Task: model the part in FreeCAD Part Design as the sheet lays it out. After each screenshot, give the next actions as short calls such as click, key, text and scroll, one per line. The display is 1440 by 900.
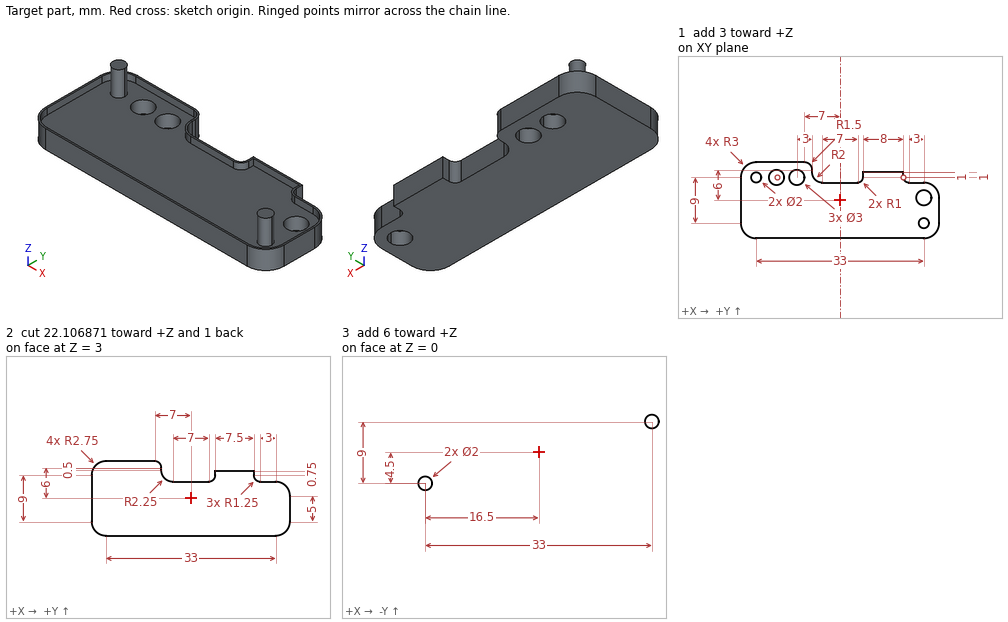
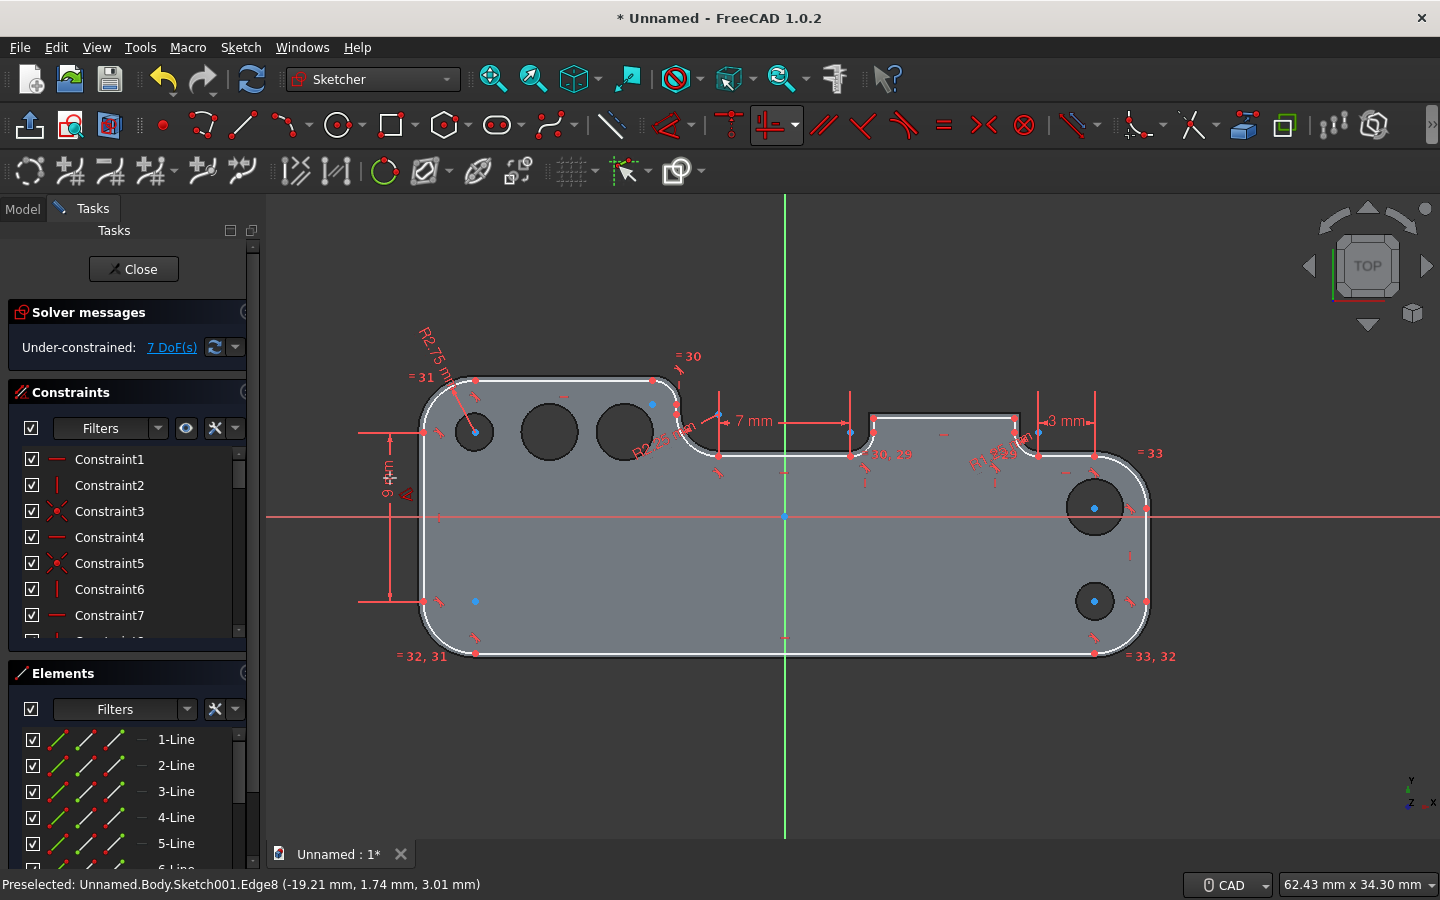
click(1147, 574)
click(1181, 555)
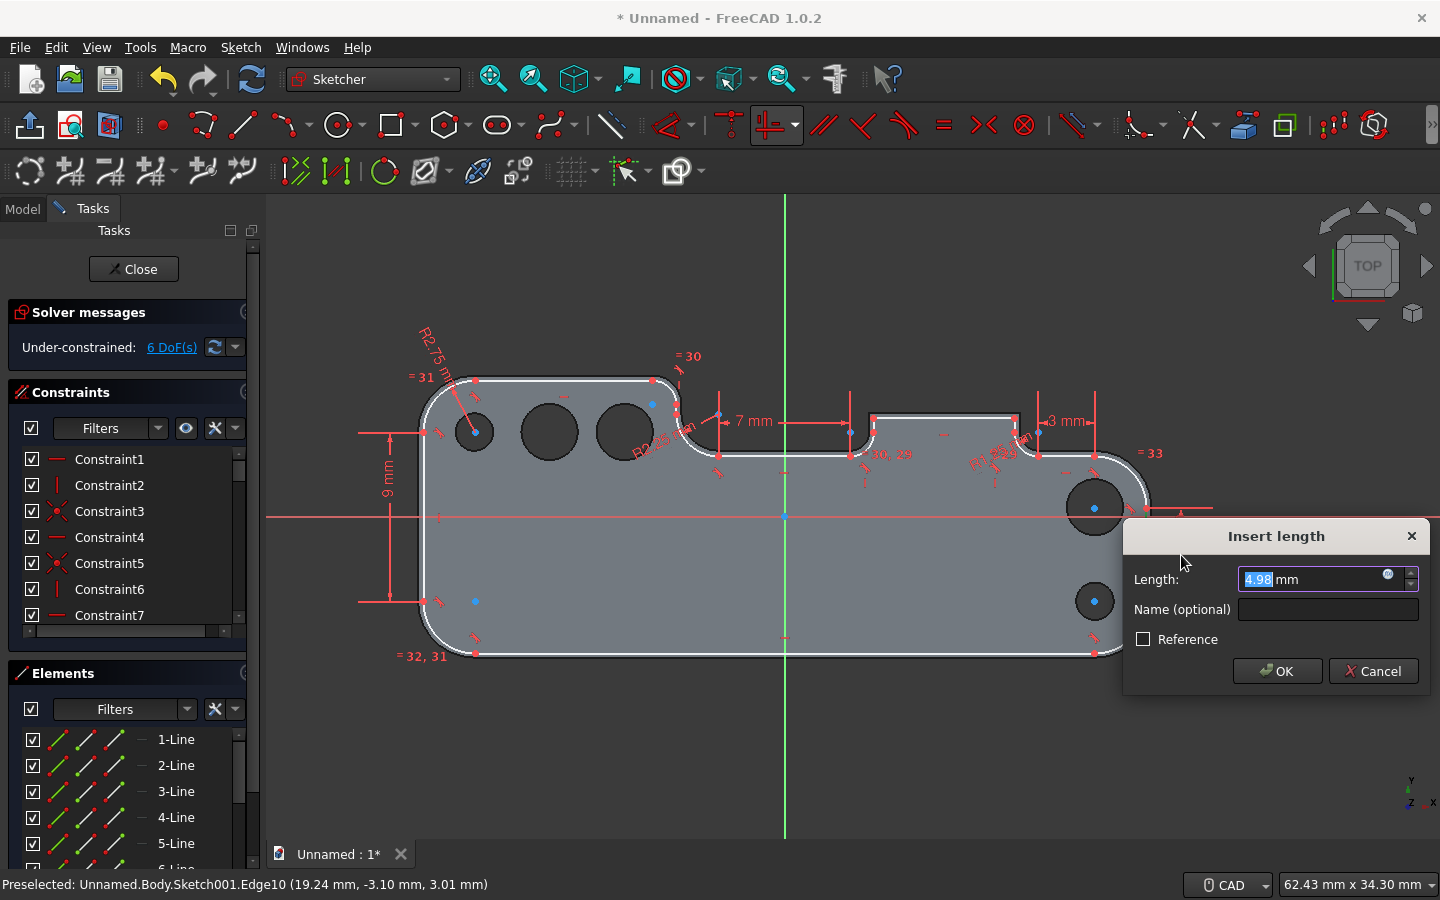
text(5)
key(Return)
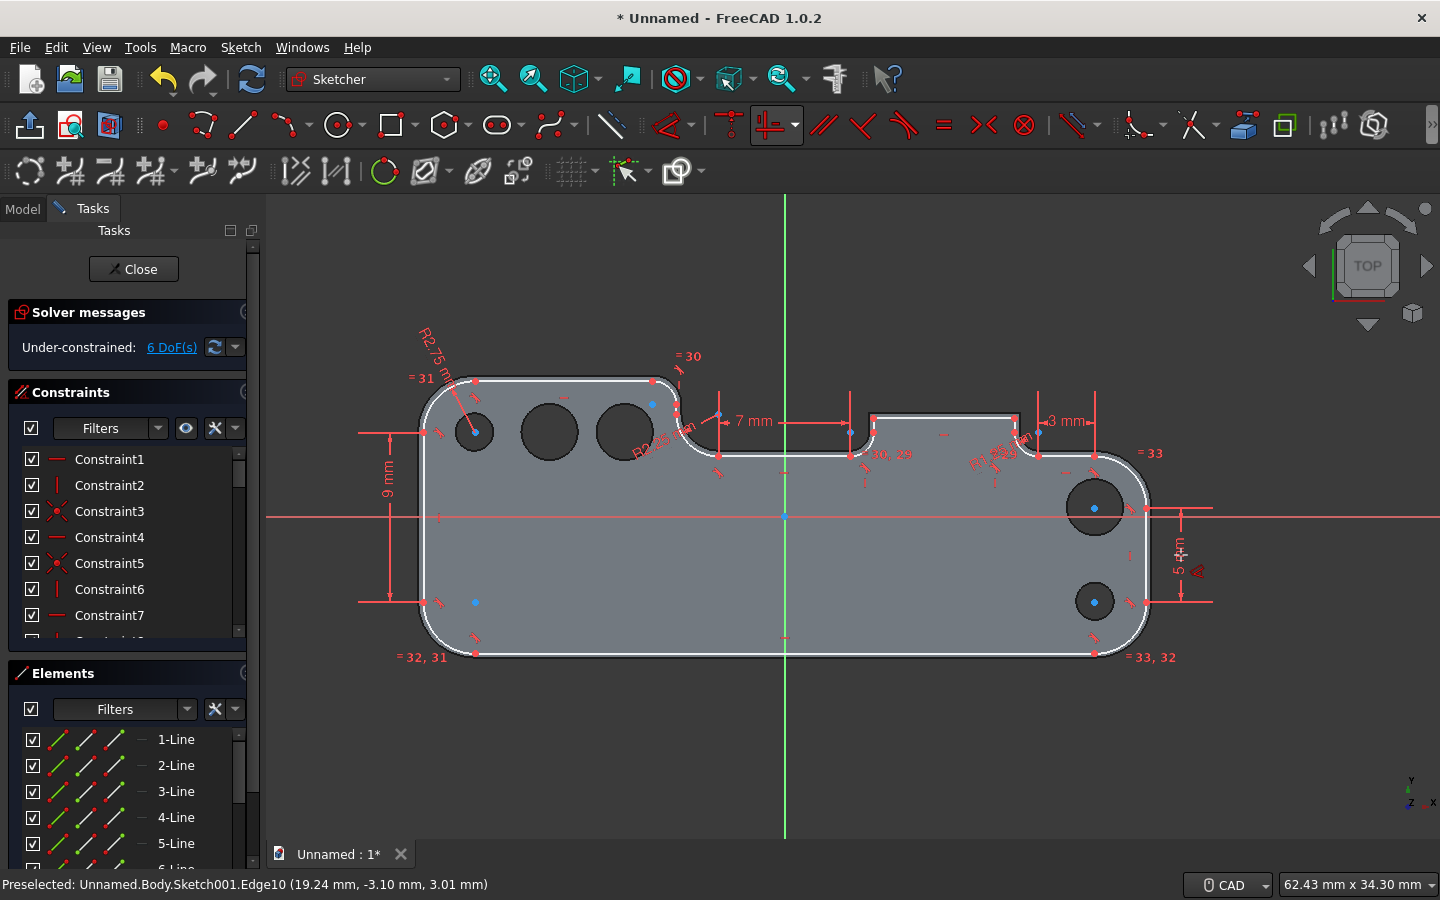
click(661, 654)
click(643, 688)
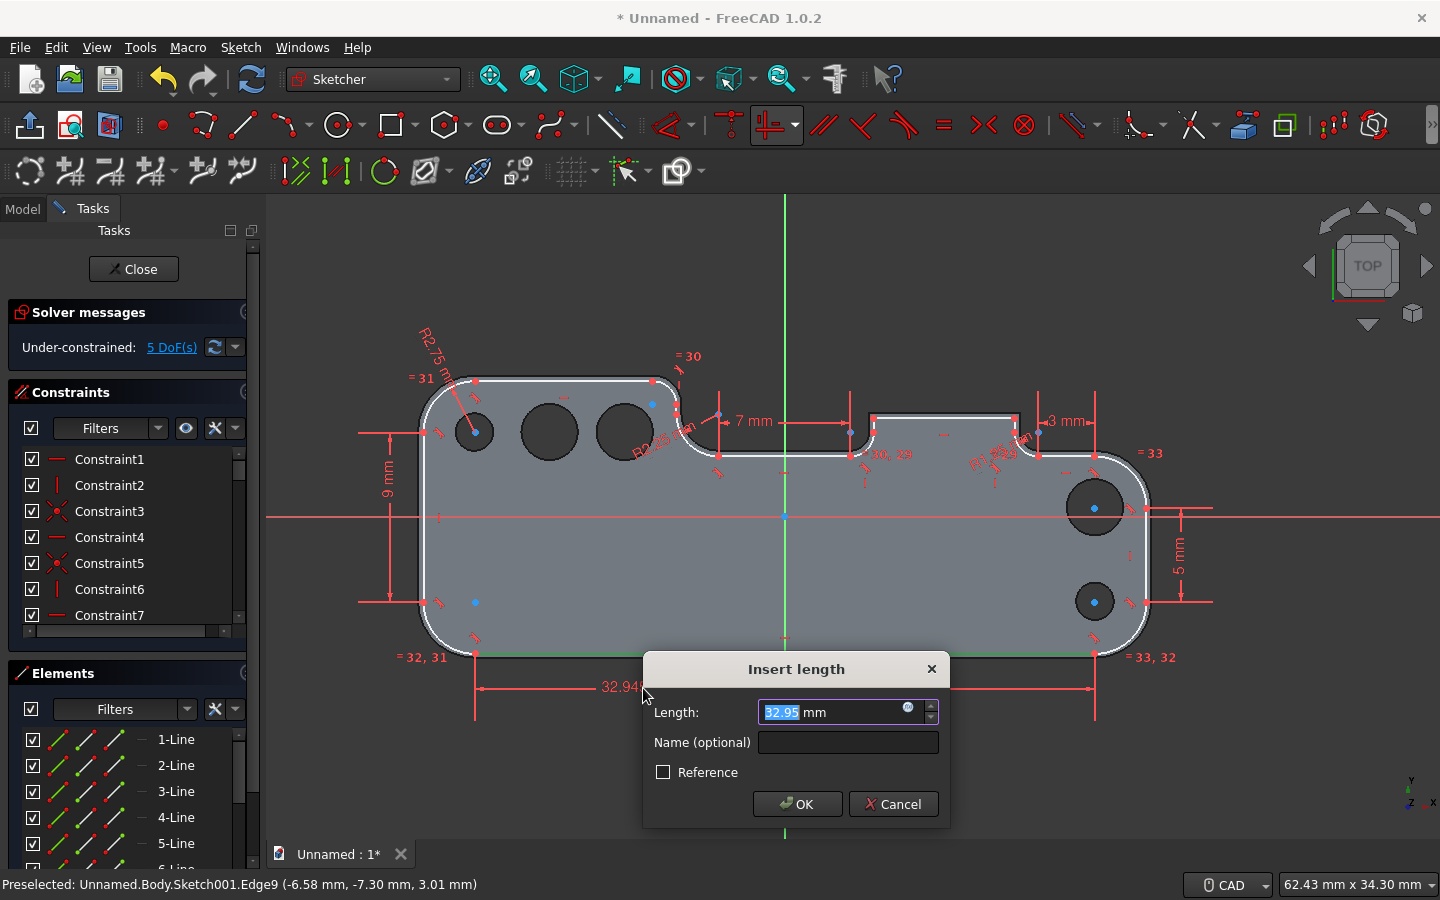
text(33)
key(Return)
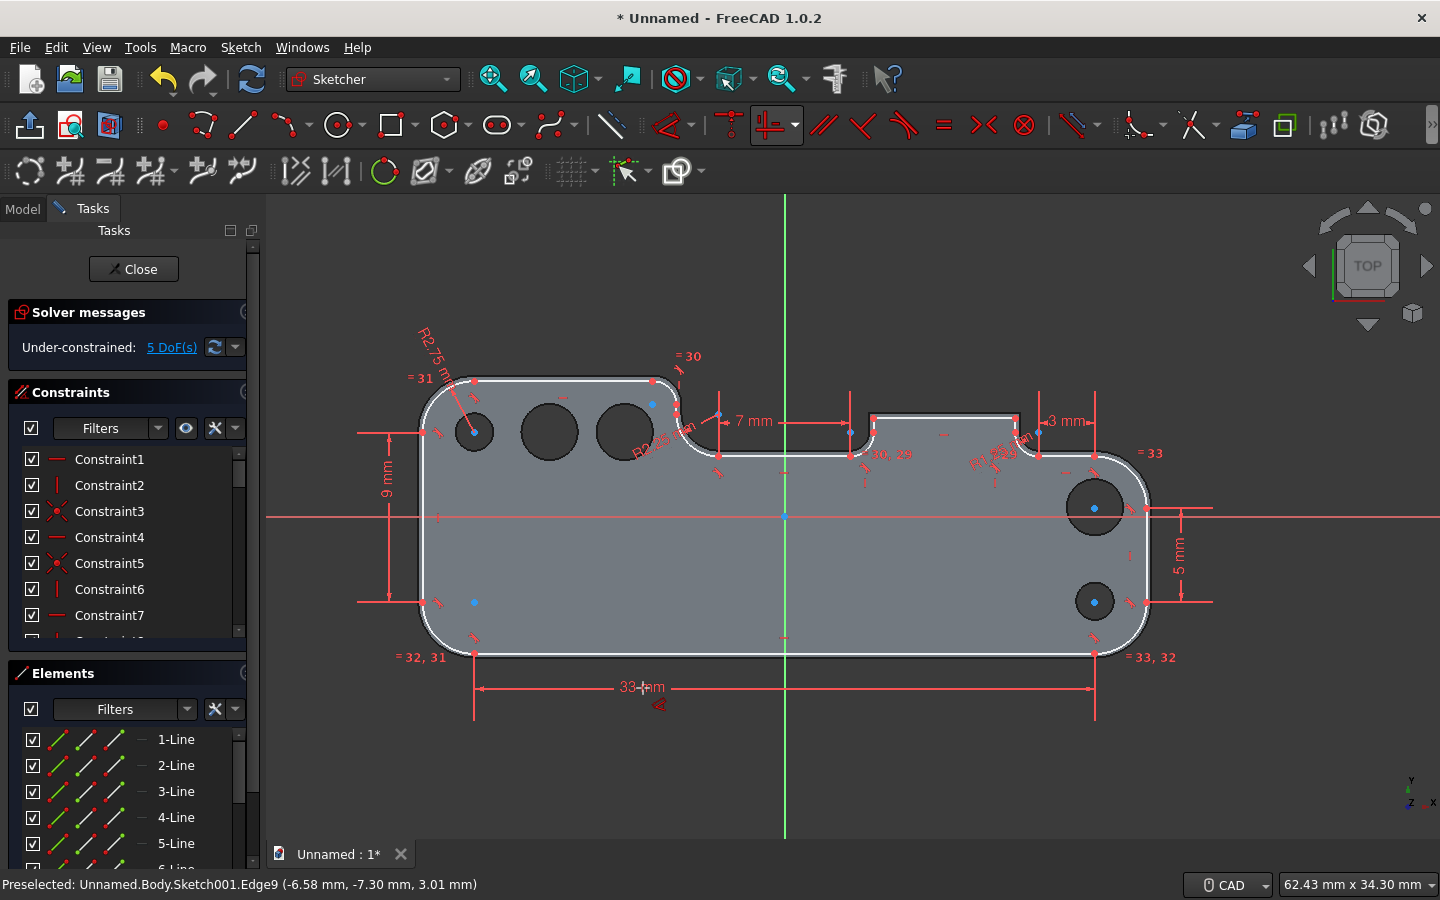
scroll(676, 405, up, 2)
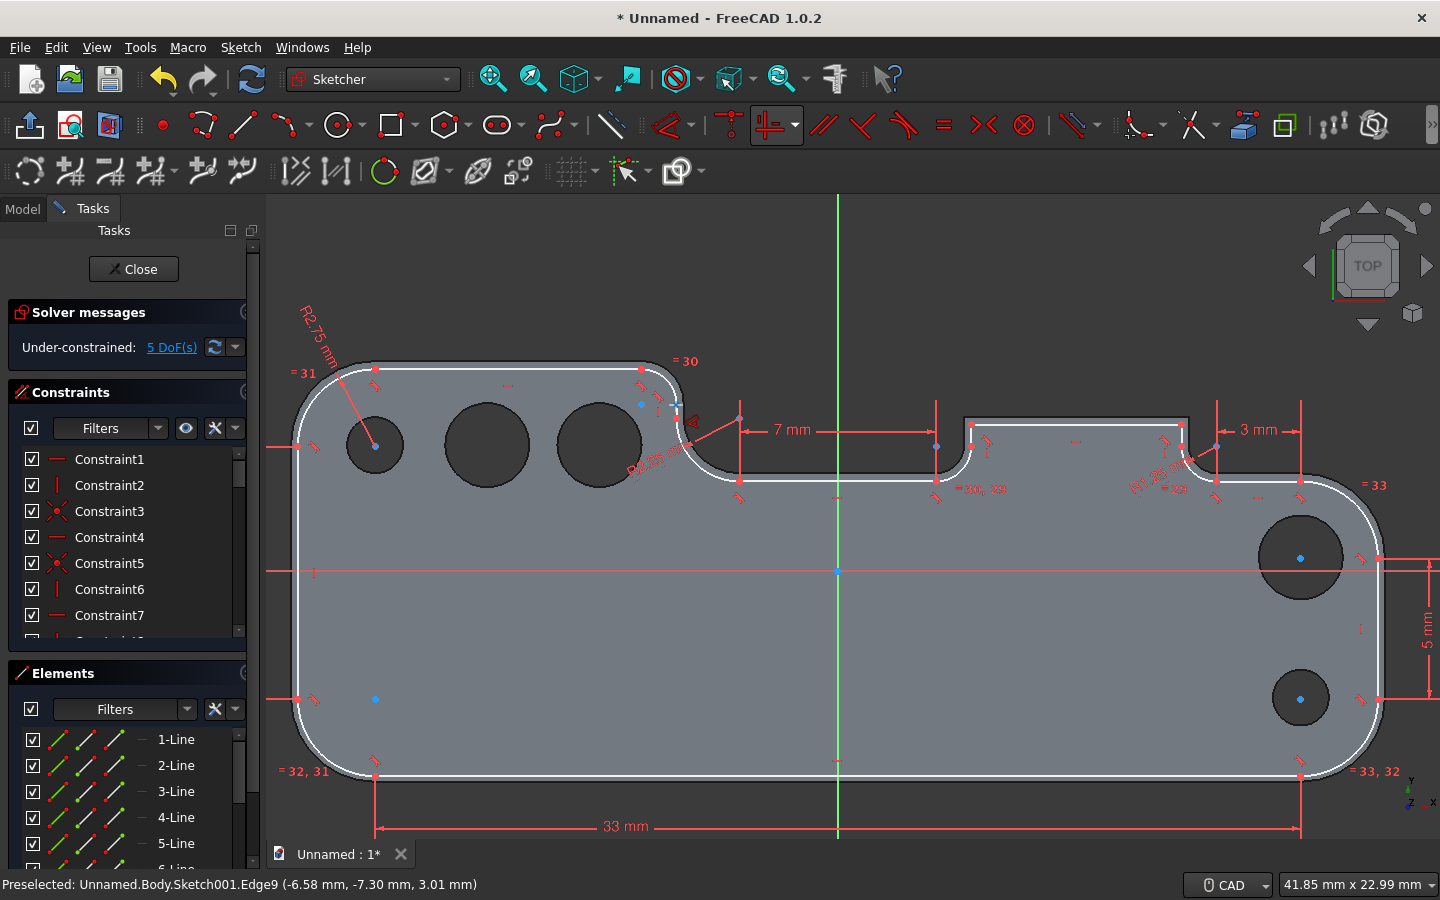
click(677, 404)
click(643, 488)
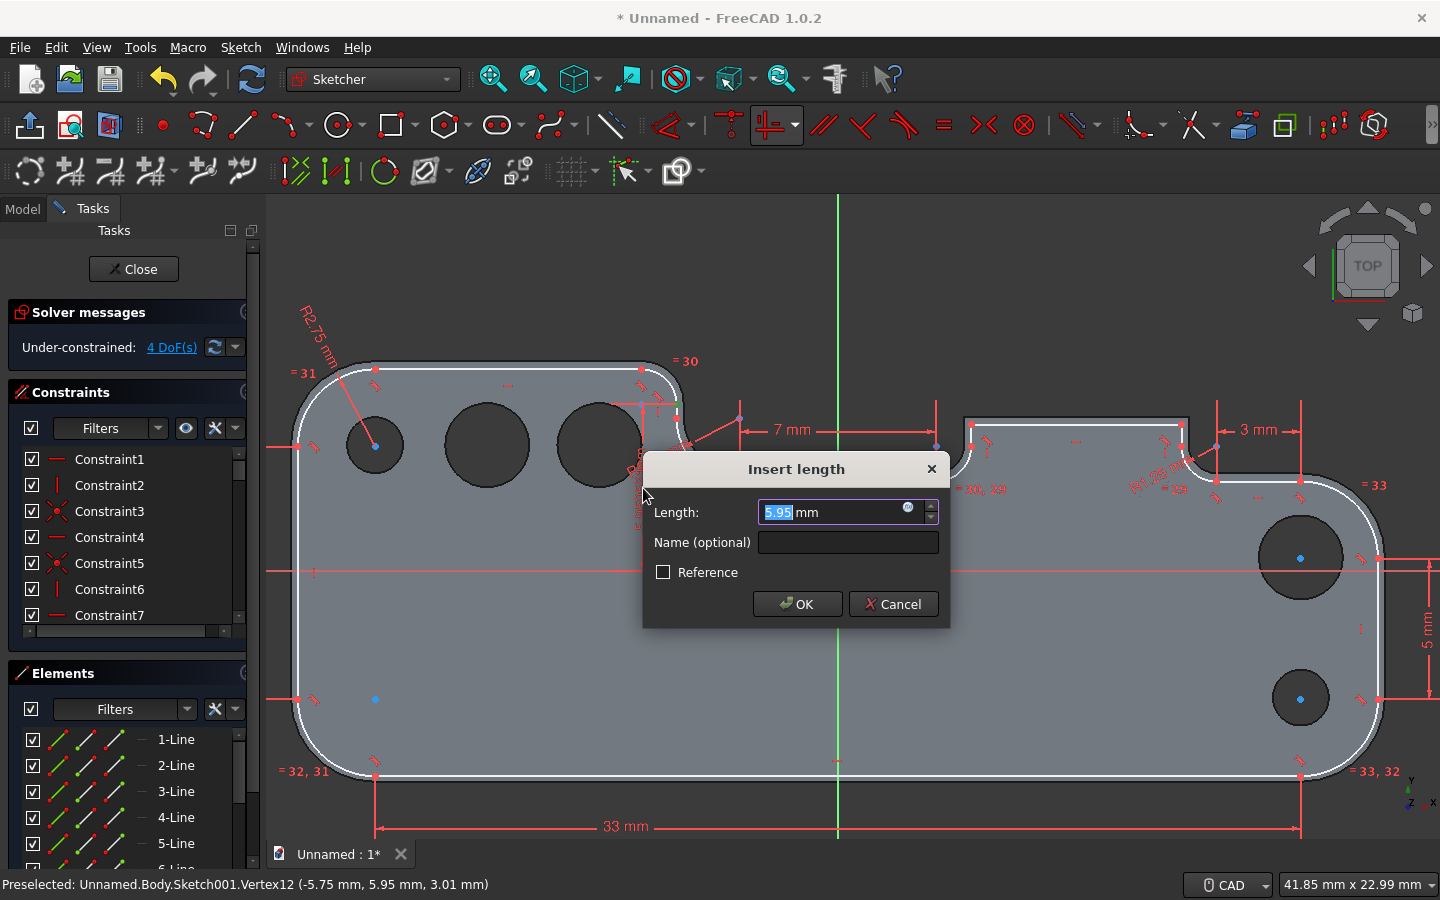
text(6)
key(Return)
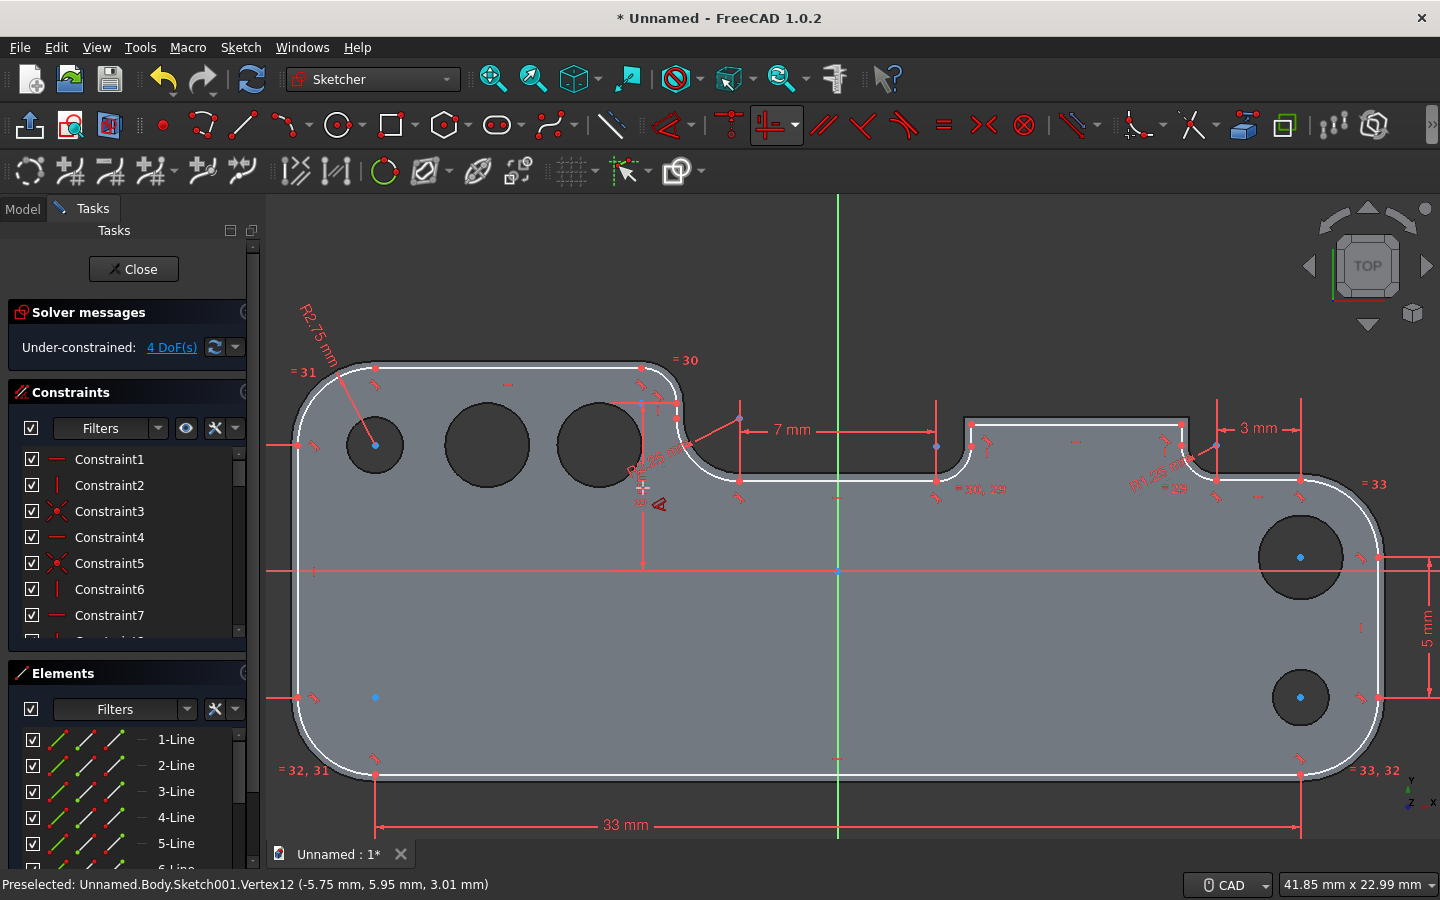
click(641, 368)
click(740, 334)